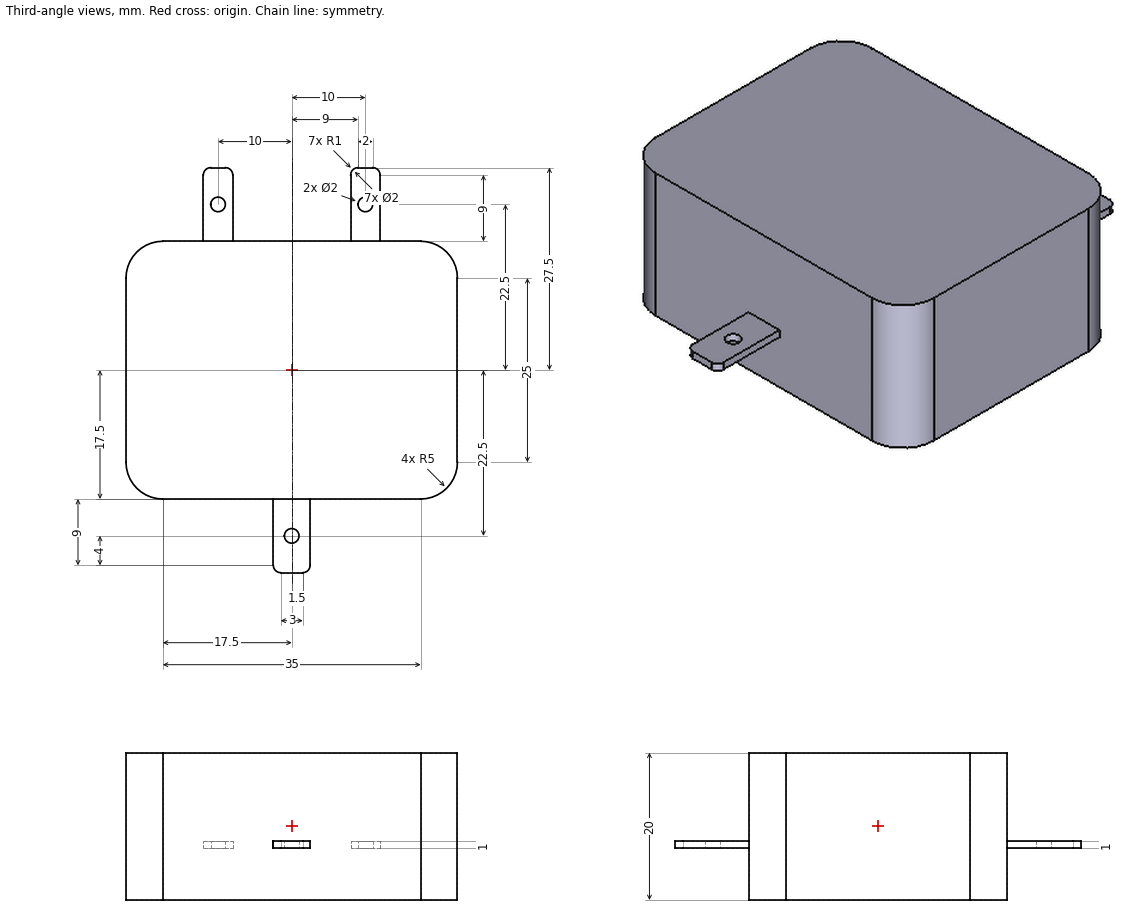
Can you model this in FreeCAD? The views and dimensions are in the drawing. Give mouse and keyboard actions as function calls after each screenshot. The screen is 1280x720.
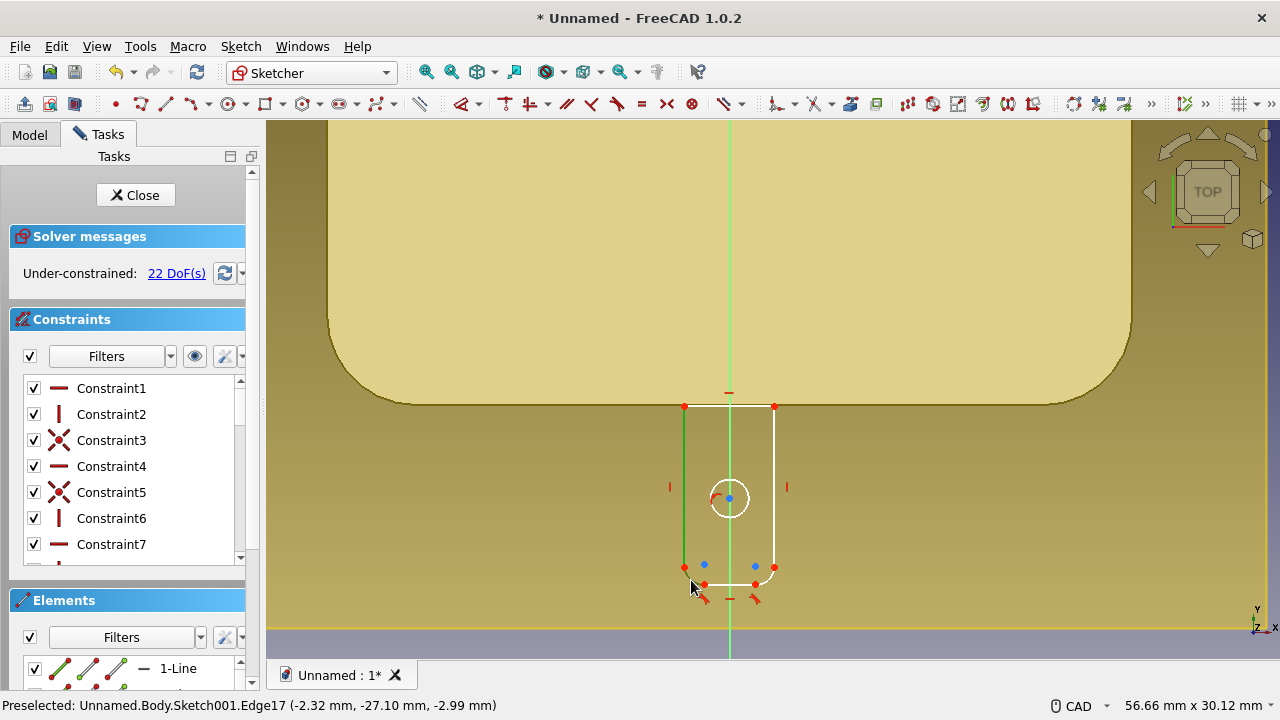
key(t)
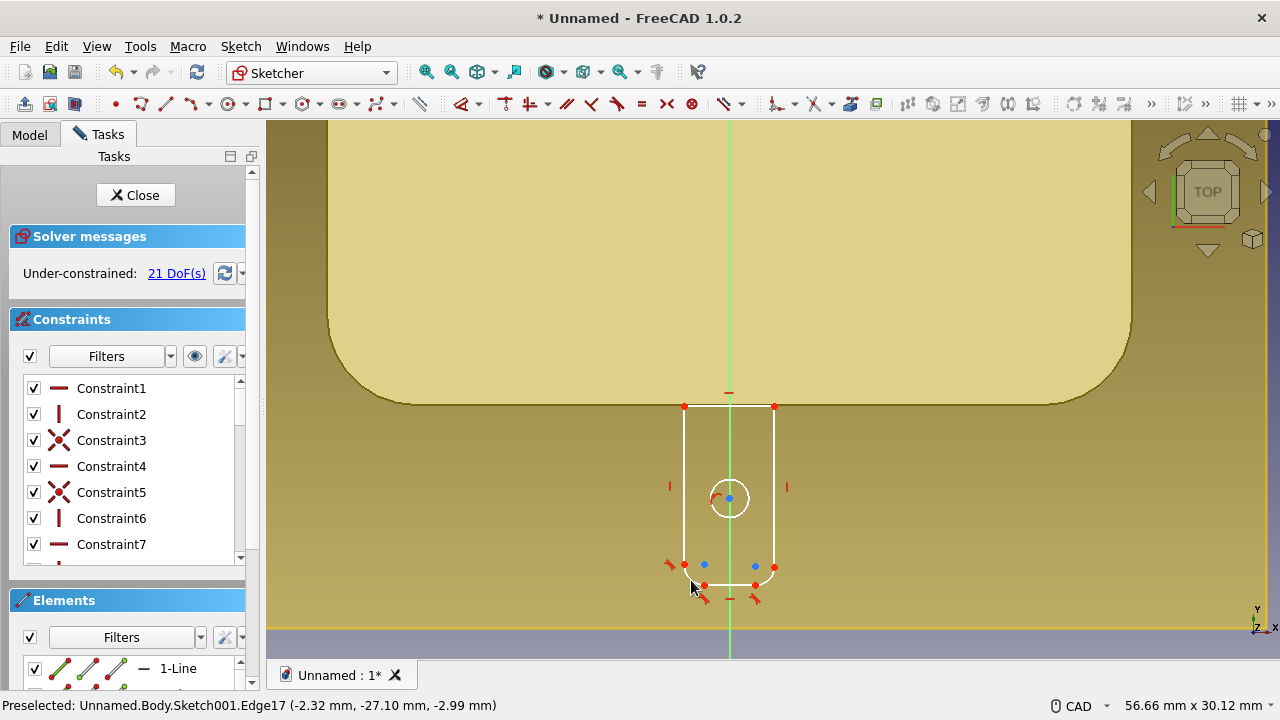
click(774, 454)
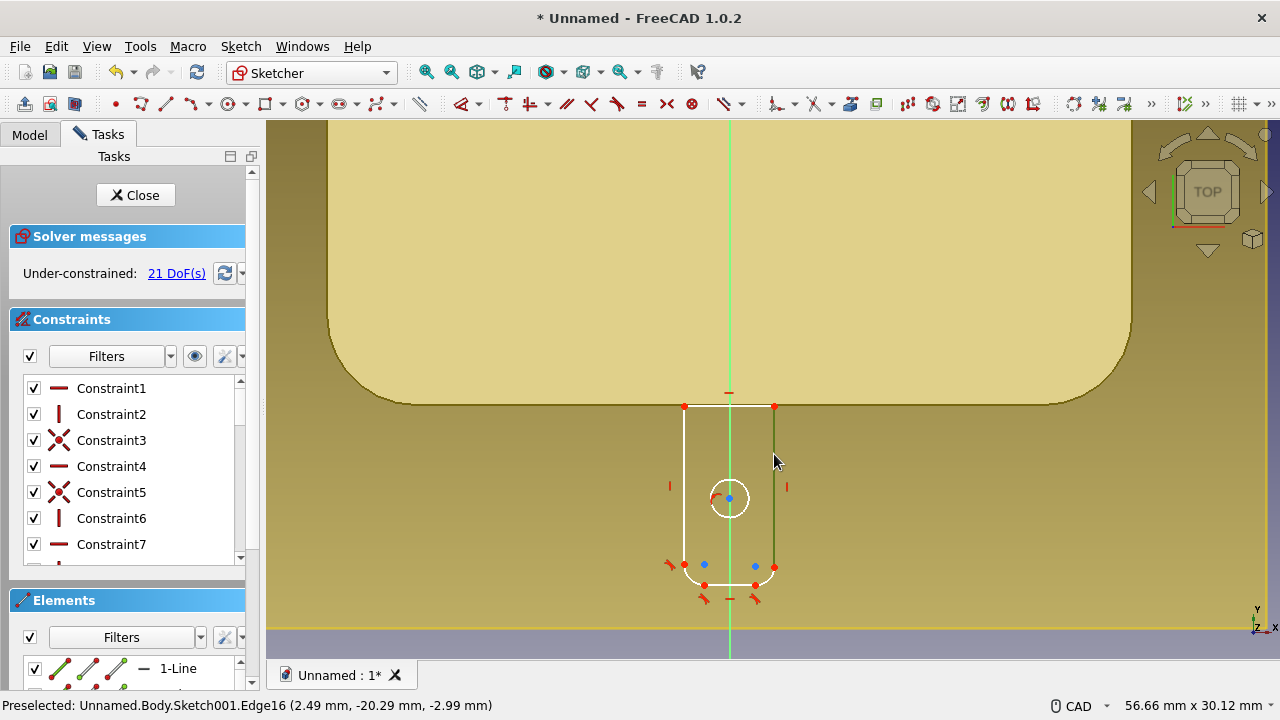
click(769, 580)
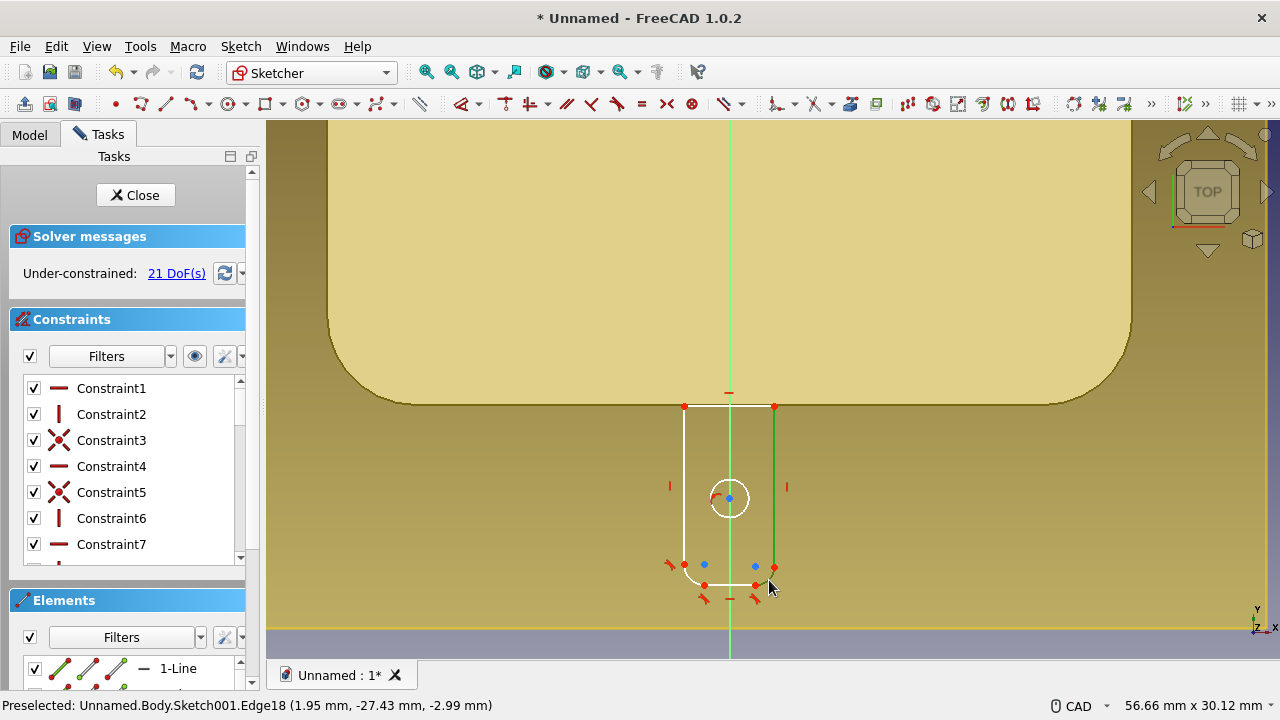
click(617, 104)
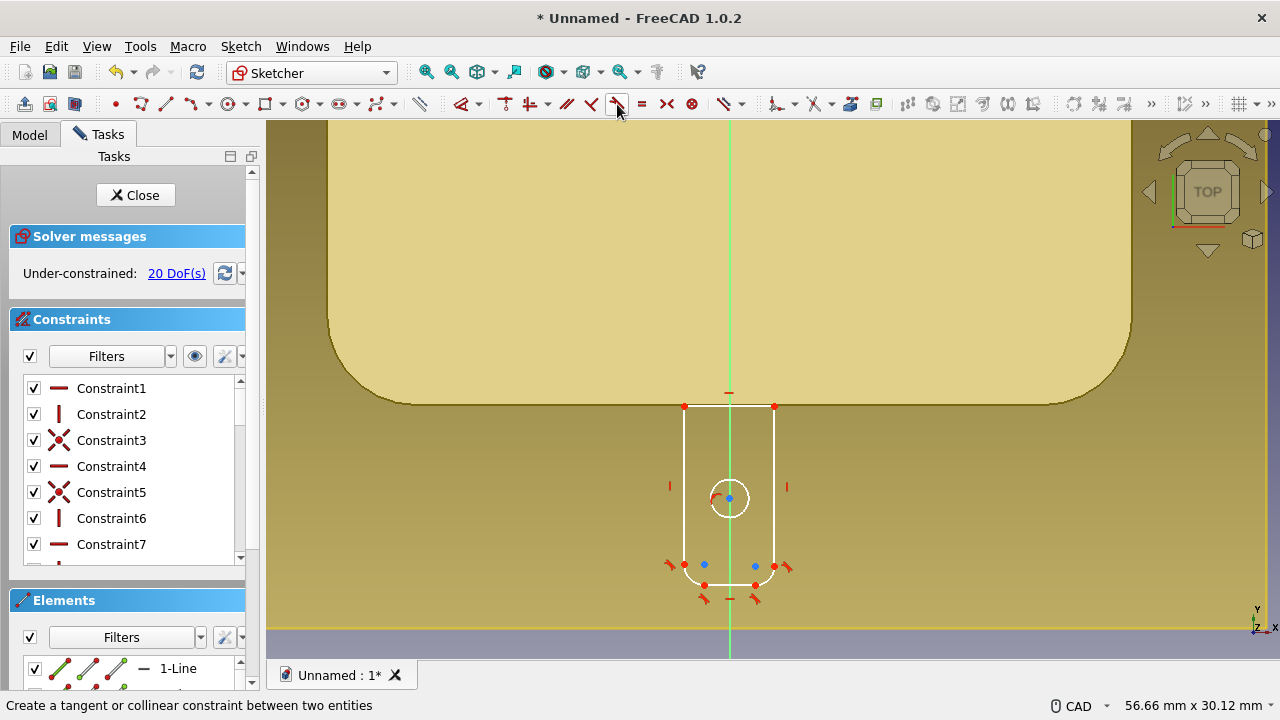
scroll(690, 563, down, 5)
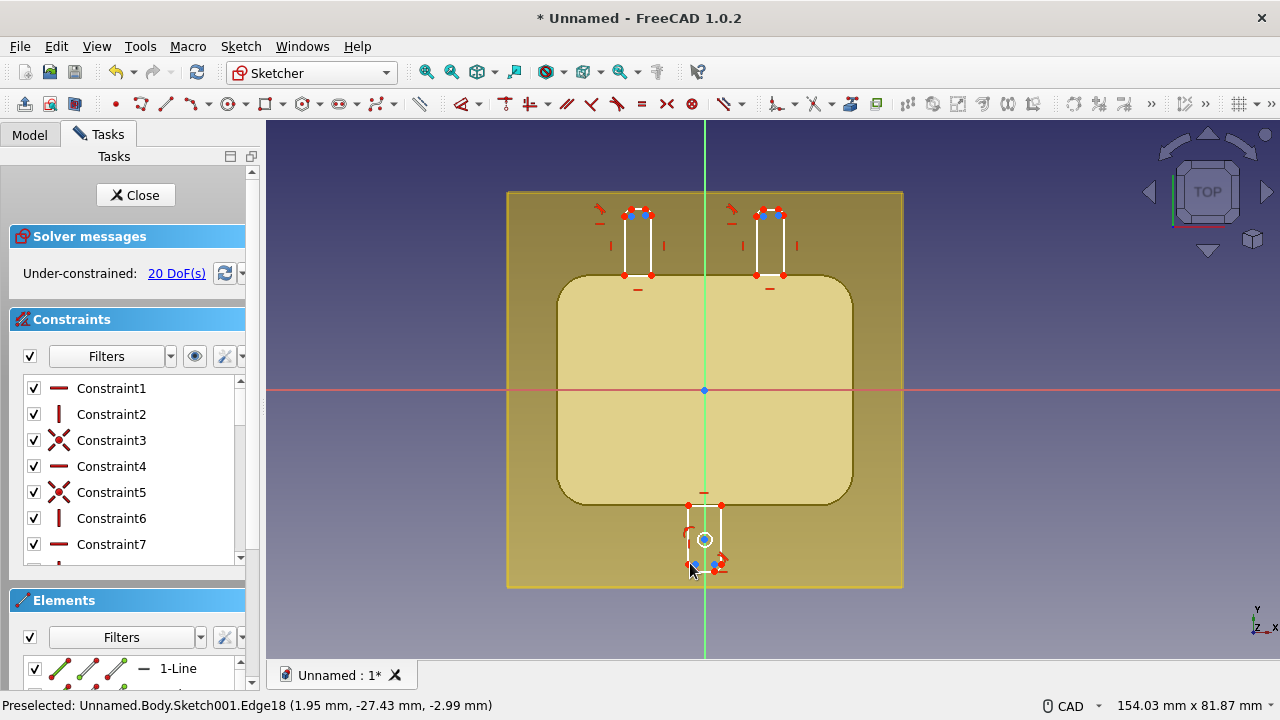
scroll(782, 212, up, 6)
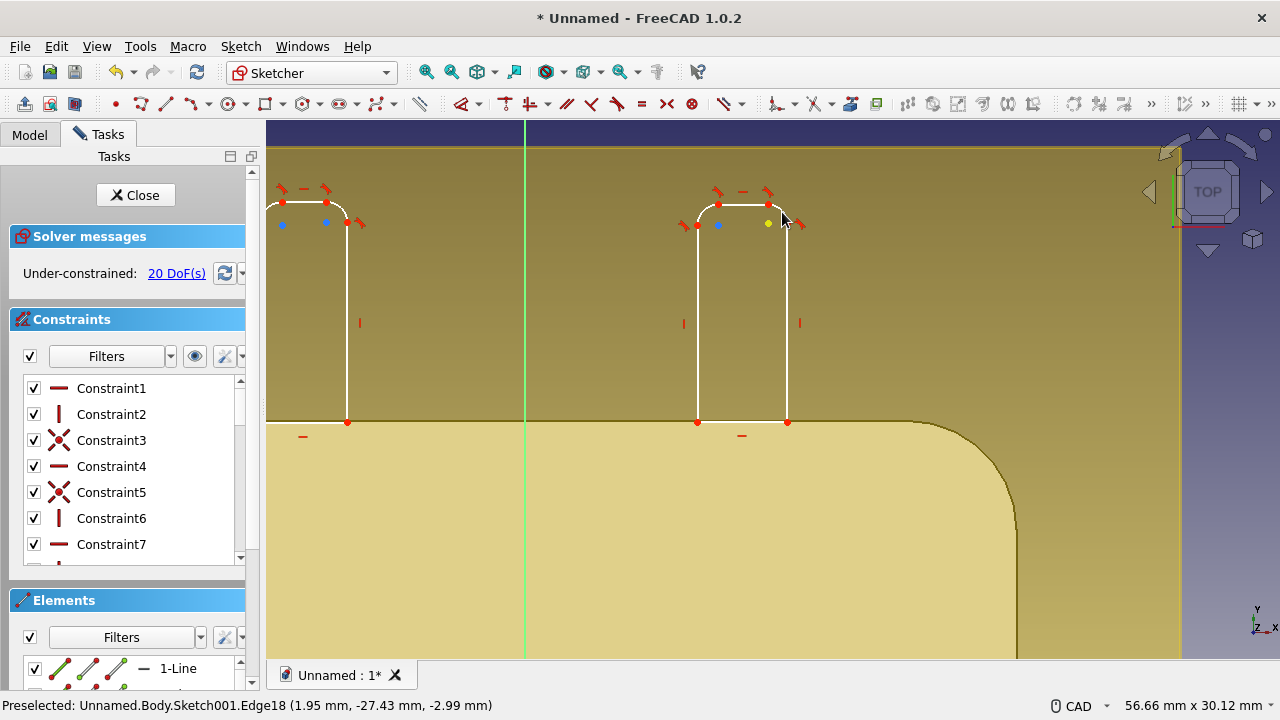
click(782, 210)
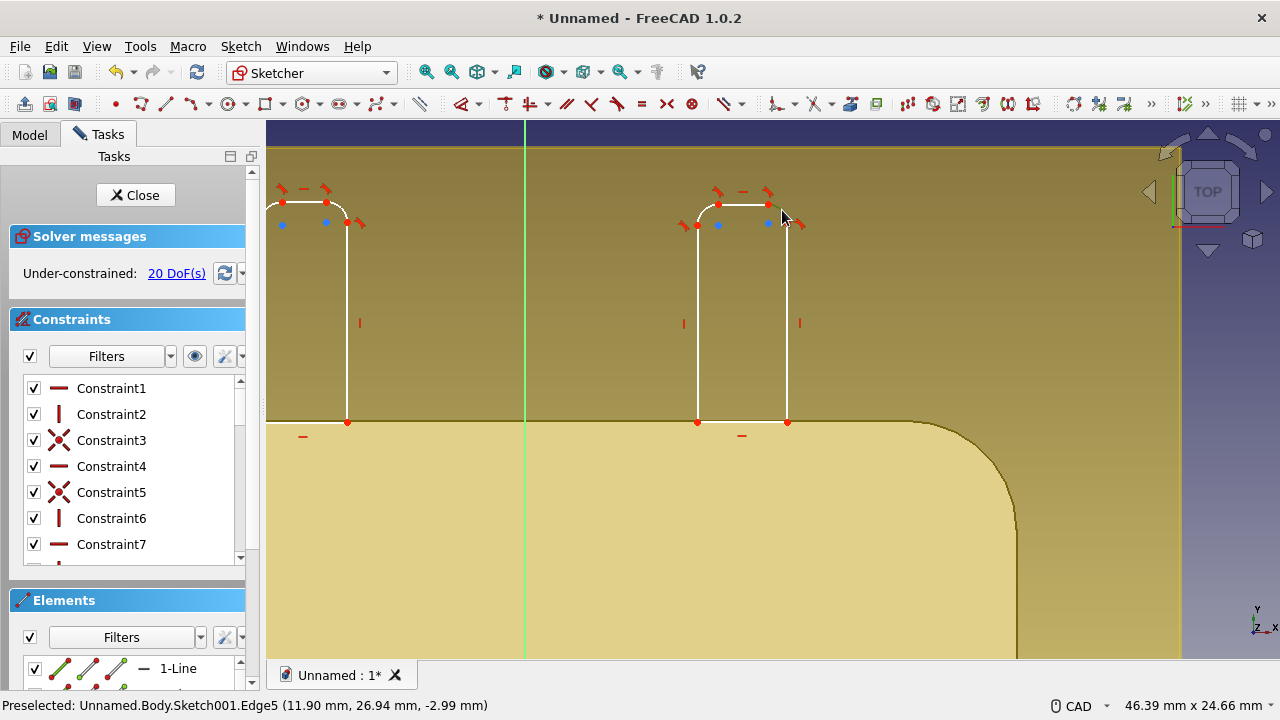
scroll(709, 207, up, 2)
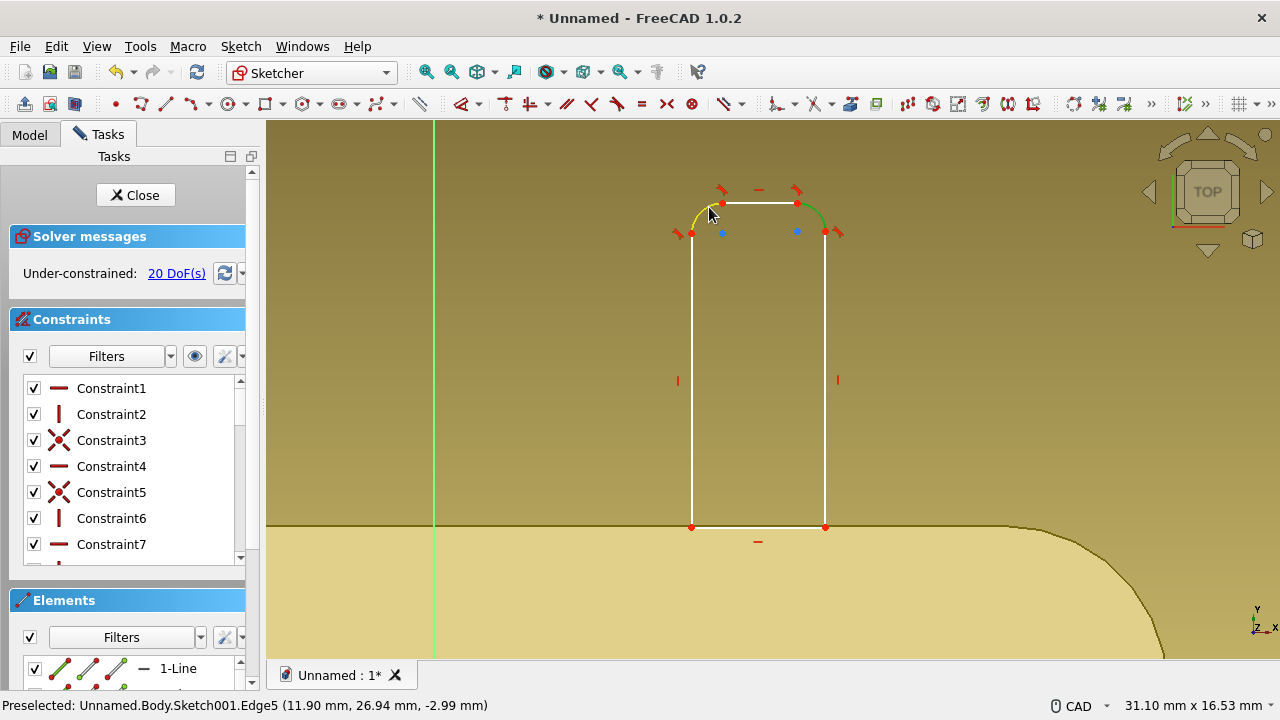
click(709, 207)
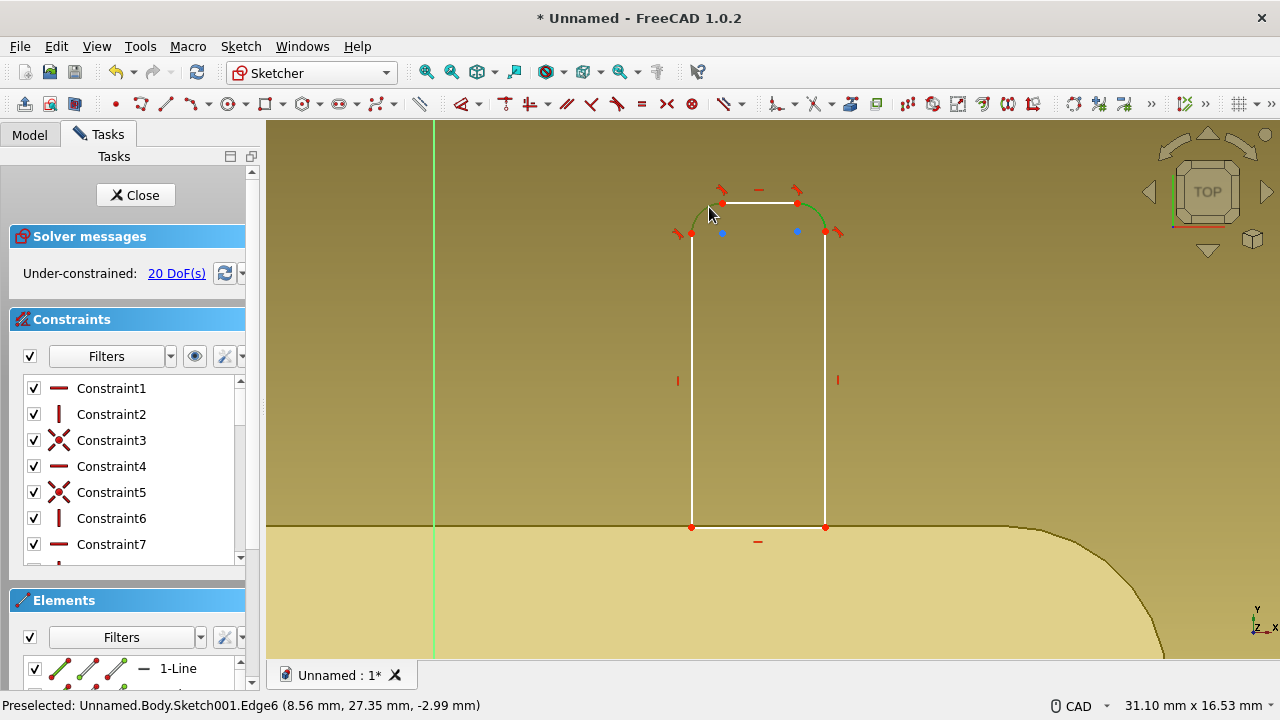
scroll(773, 211, down, 8)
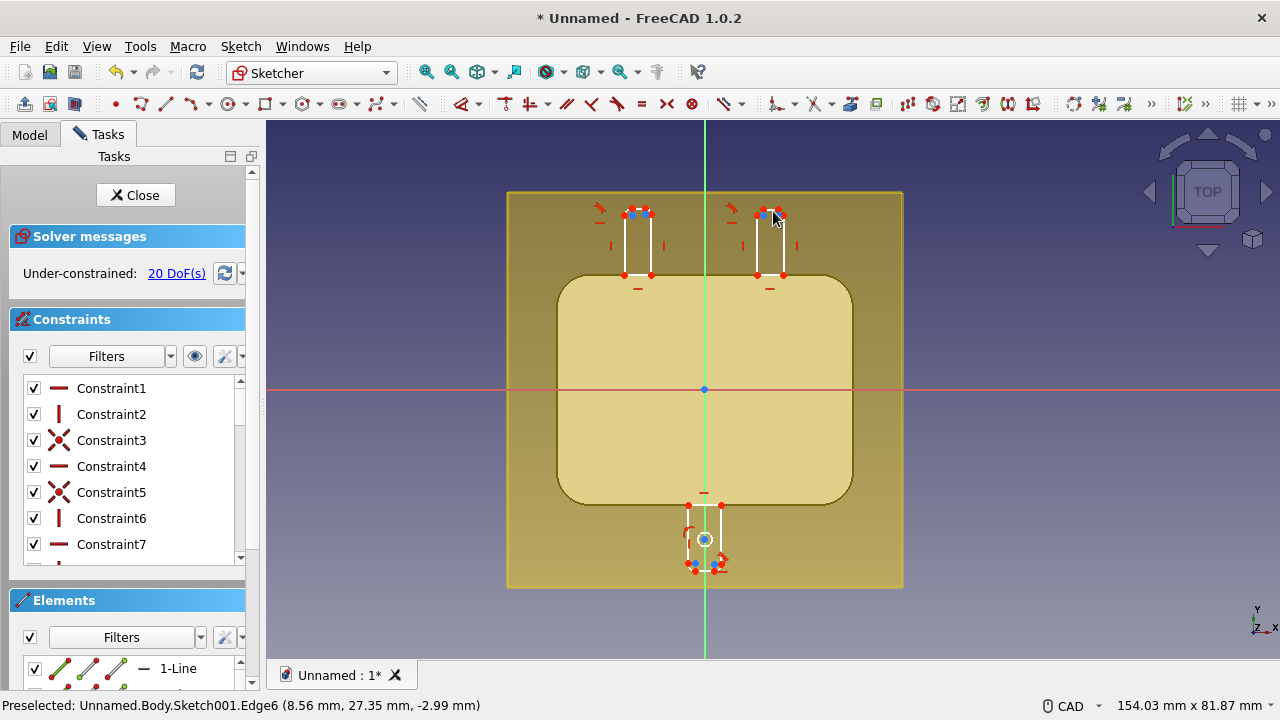
scroll(651, 212, up, 8)